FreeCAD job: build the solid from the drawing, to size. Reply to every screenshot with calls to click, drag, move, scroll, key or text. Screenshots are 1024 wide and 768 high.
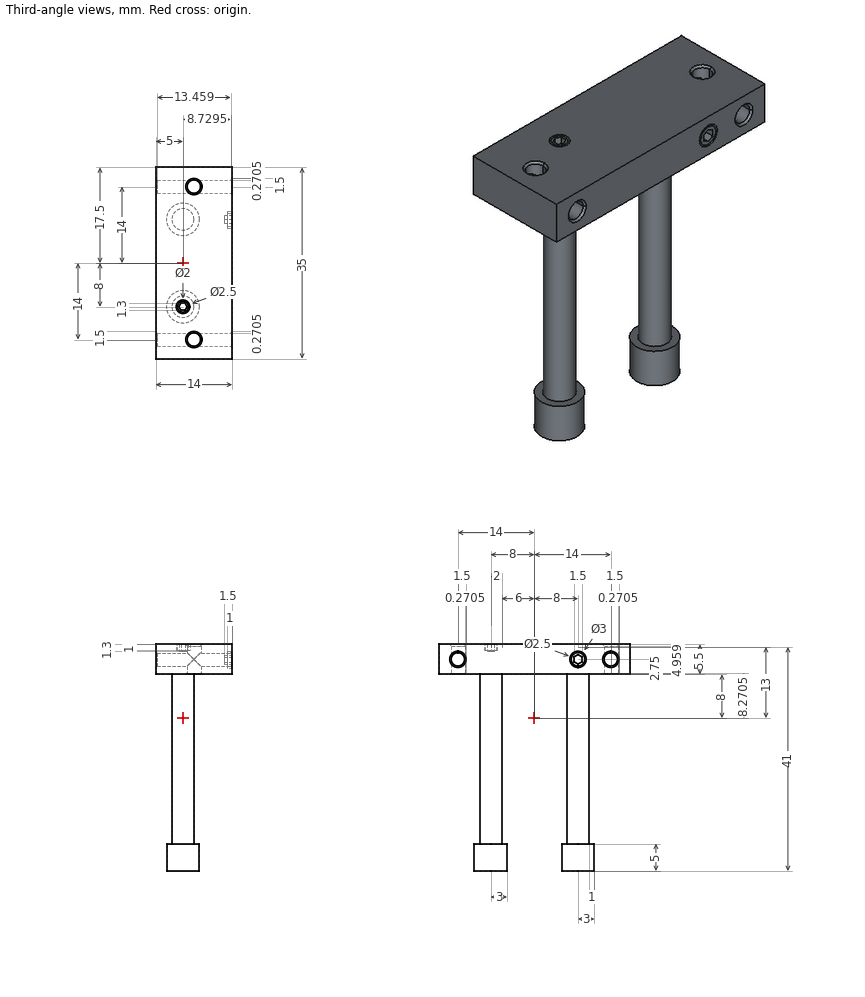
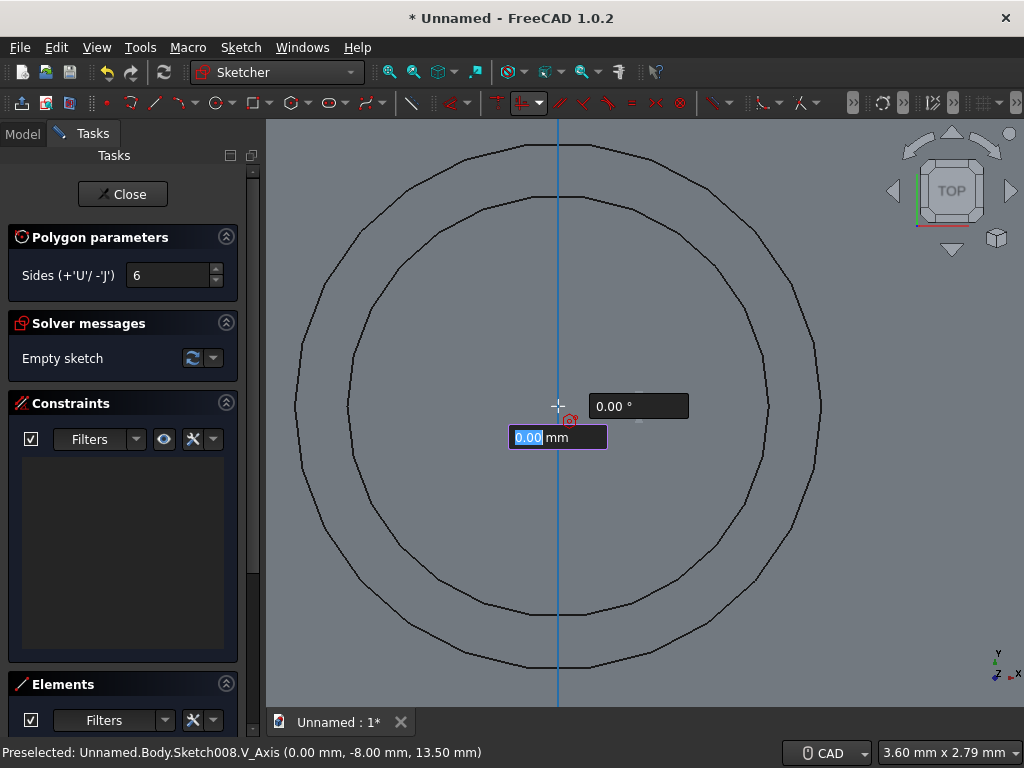
click(400, 406)
right_click(400, 406)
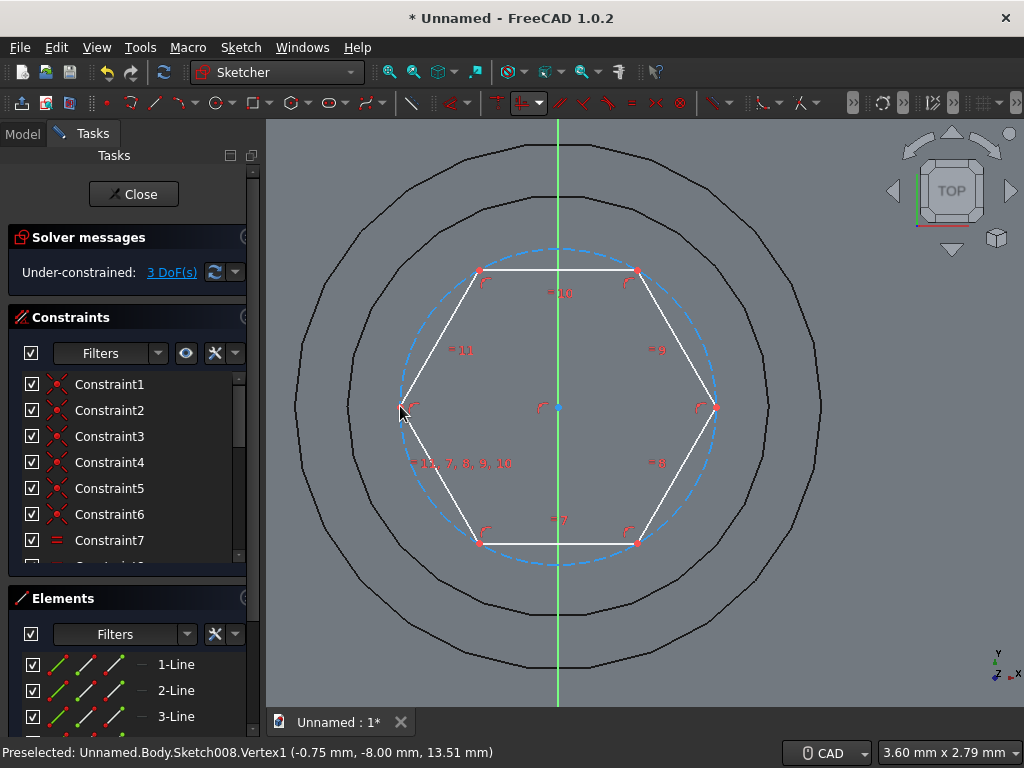
click(527, 544)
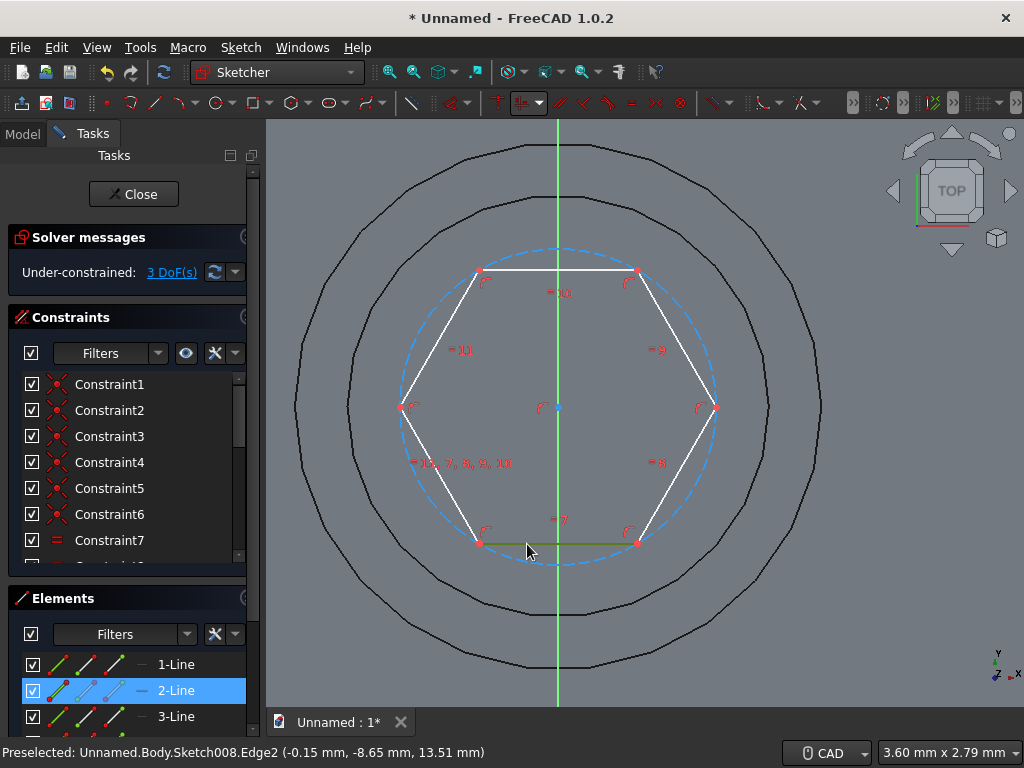
click(542, 104)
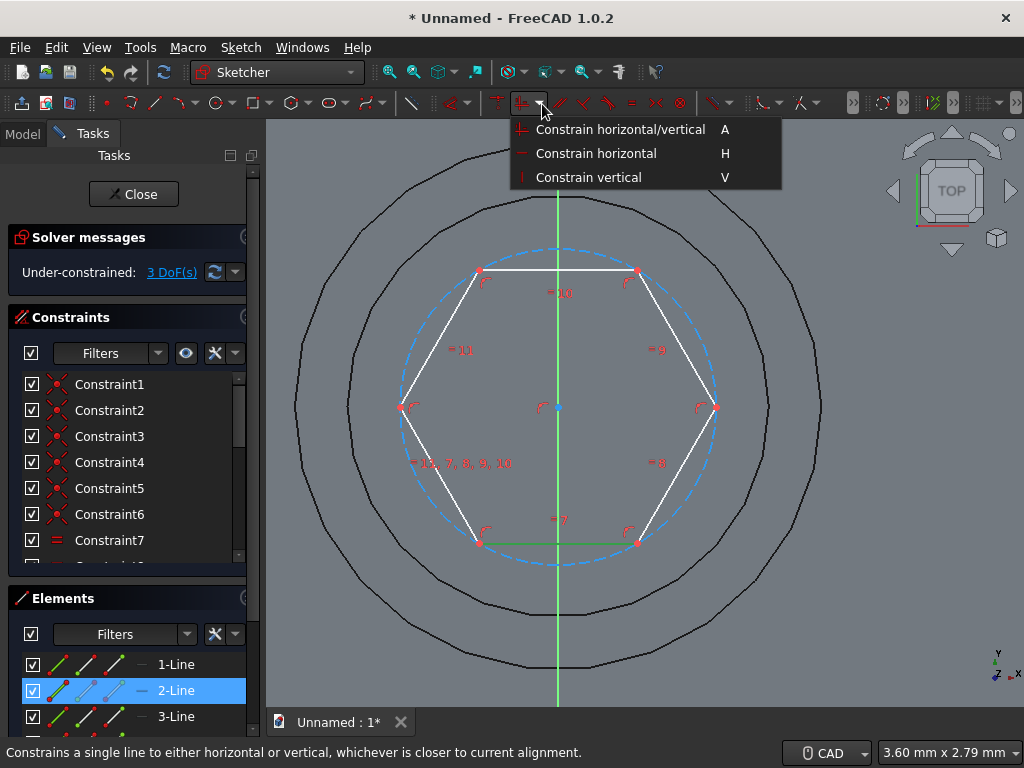
click(646, 153)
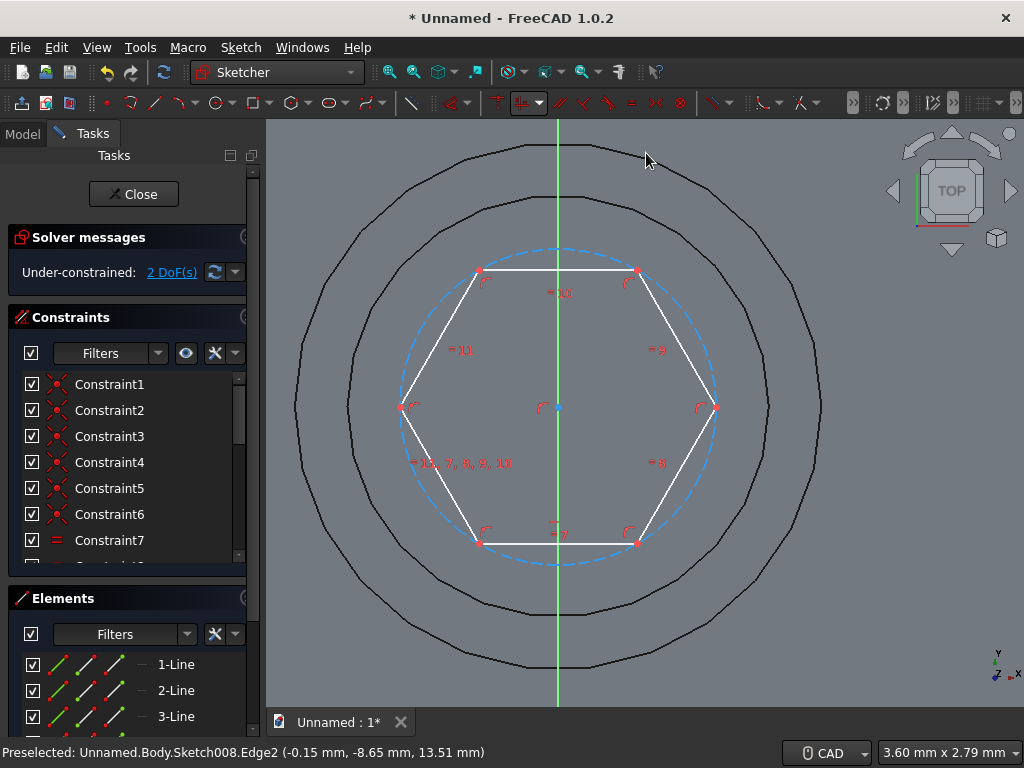
click(450, 104)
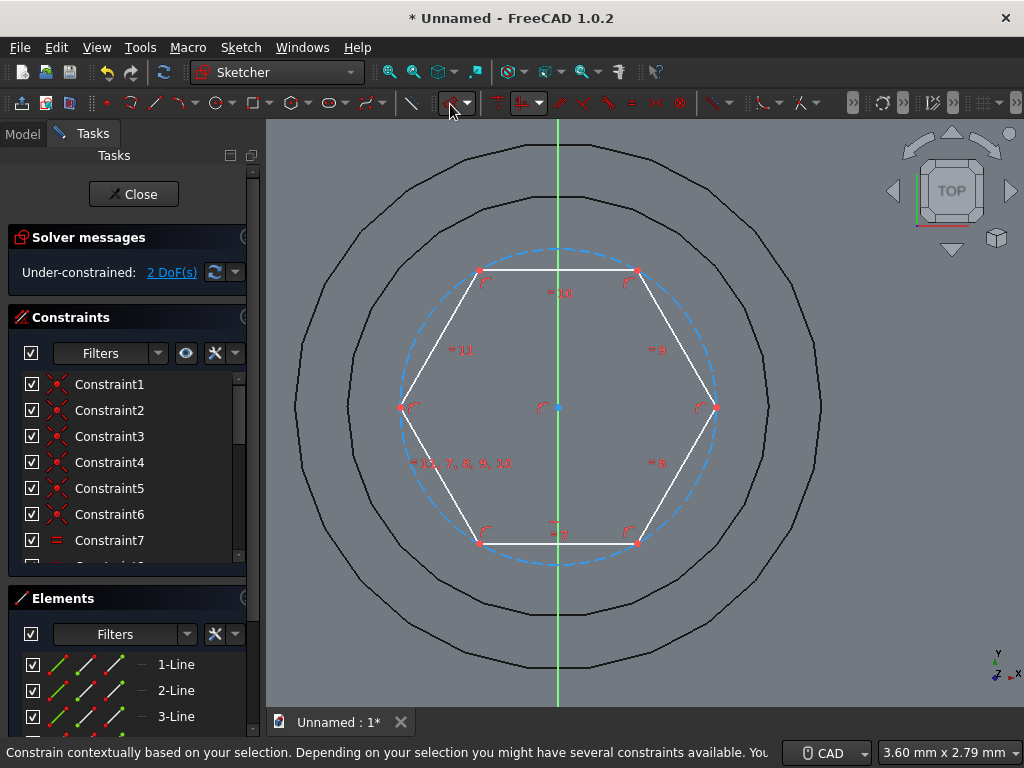
click(558, 407)
click(592, 217)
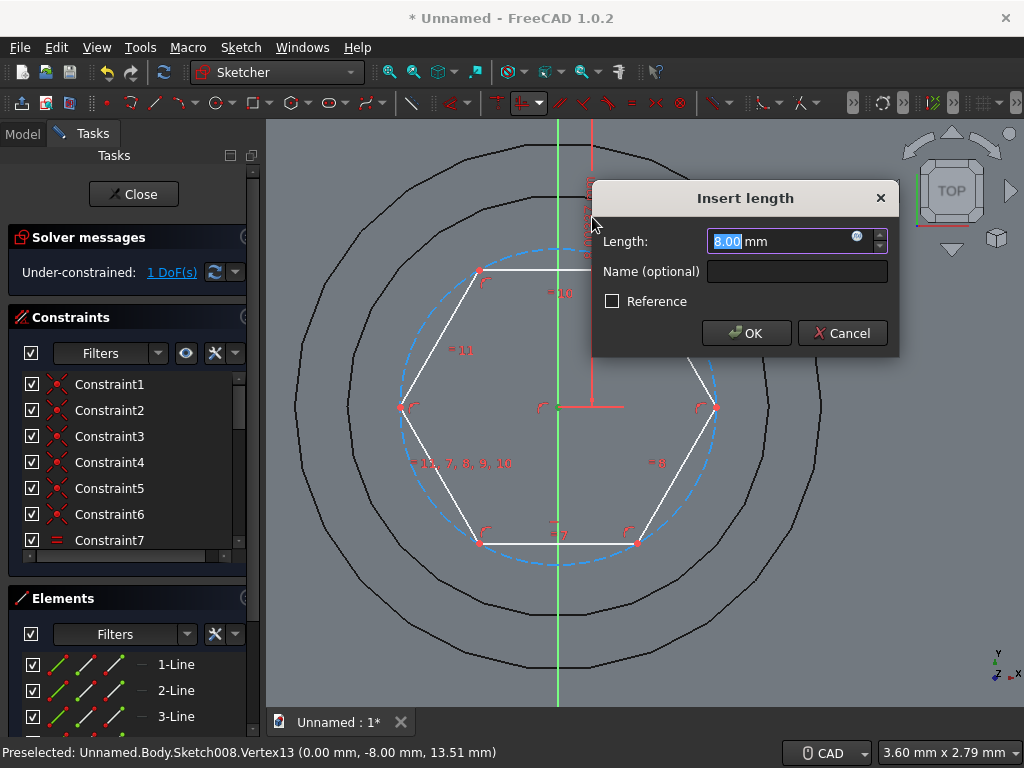
text(8)
key(Return)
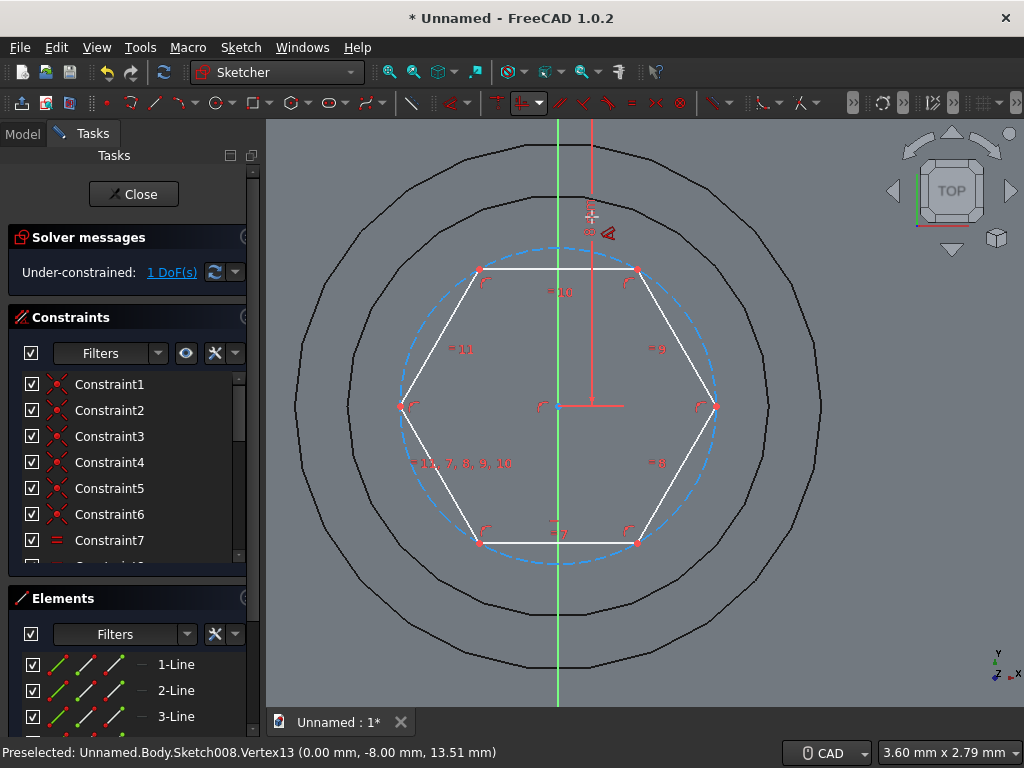
click(479, 543)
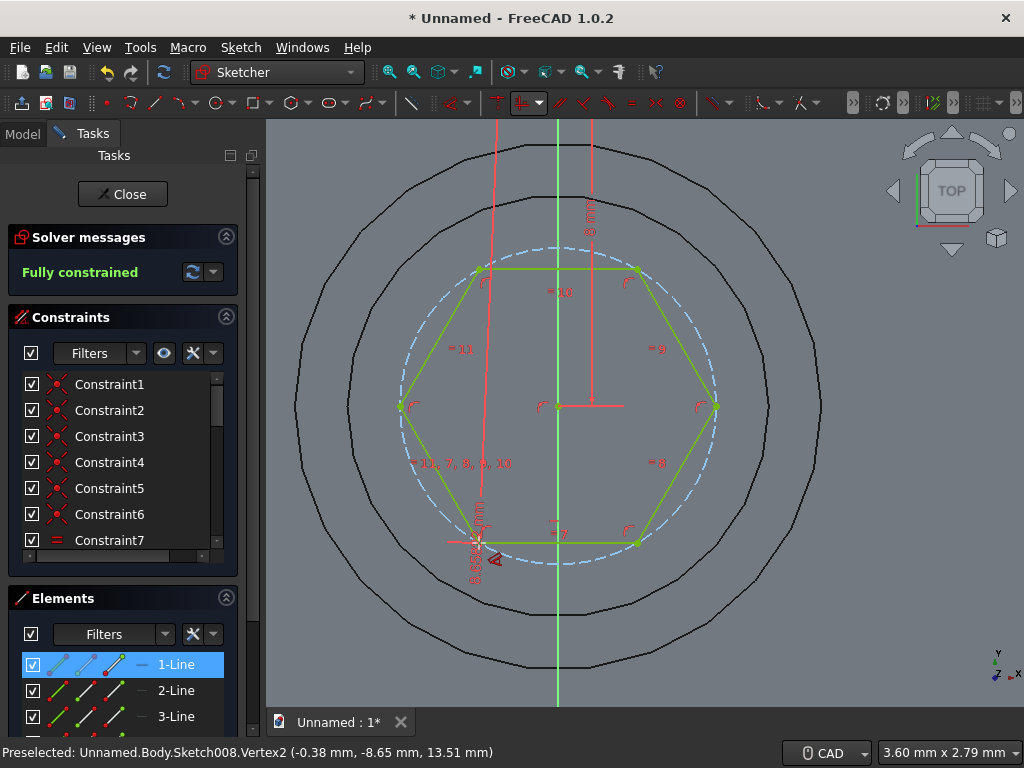
click(637, 269)
click(445, 406)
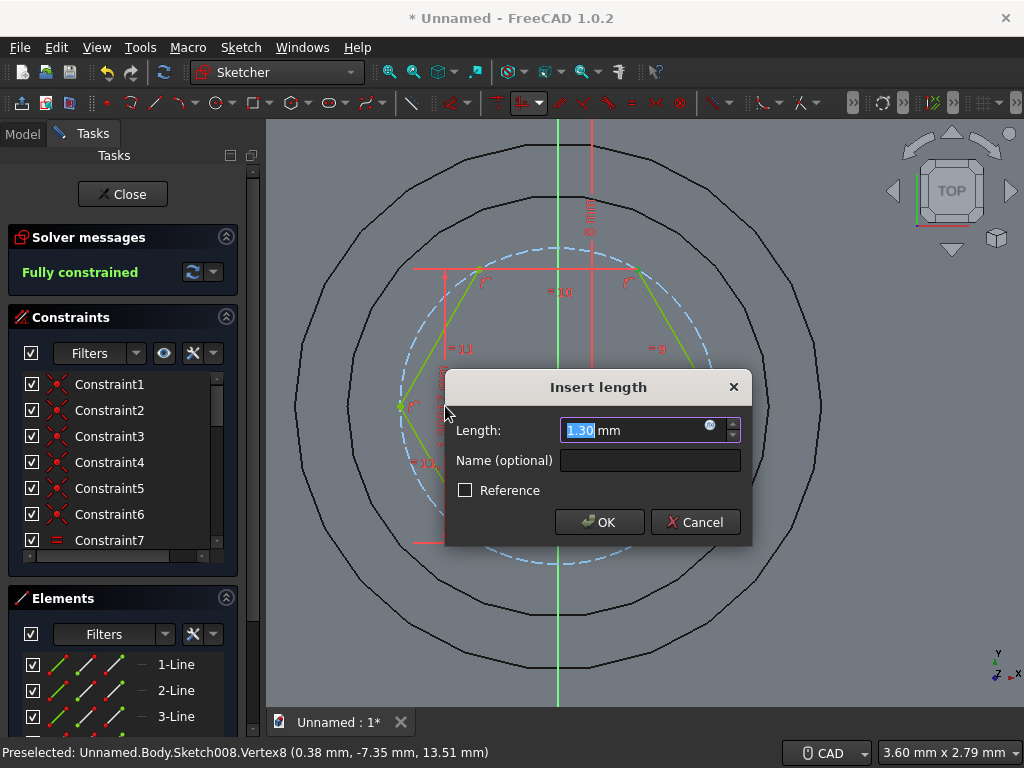
text(1.3)
key(Return)
key(Escape)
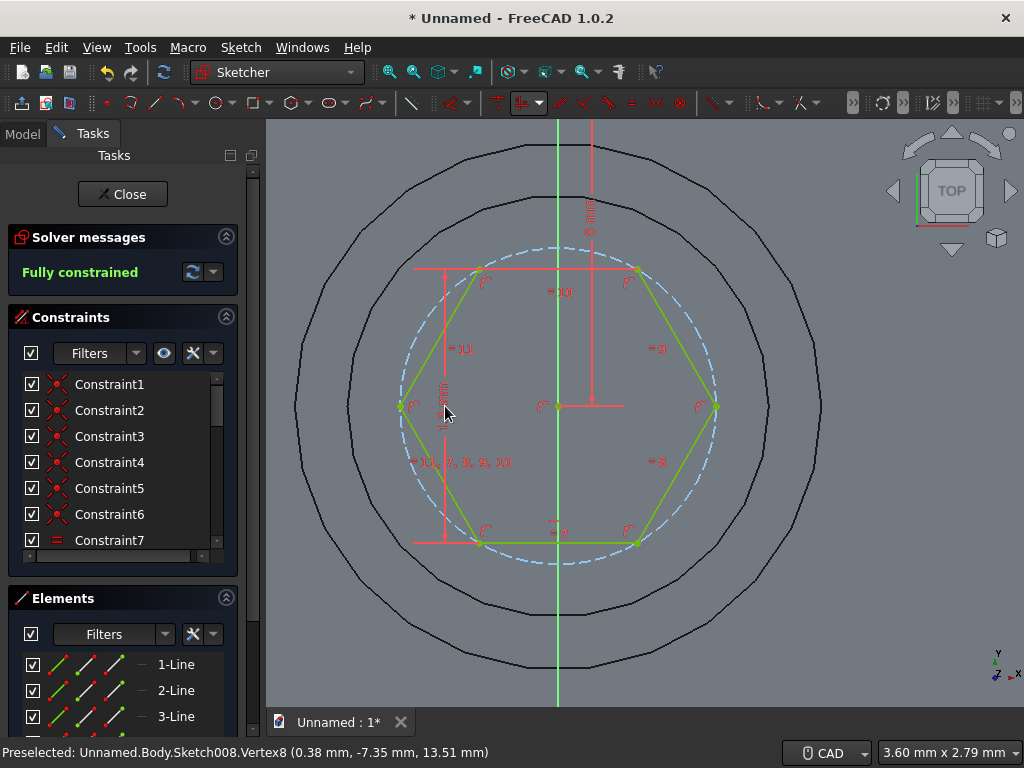
click(123, 194)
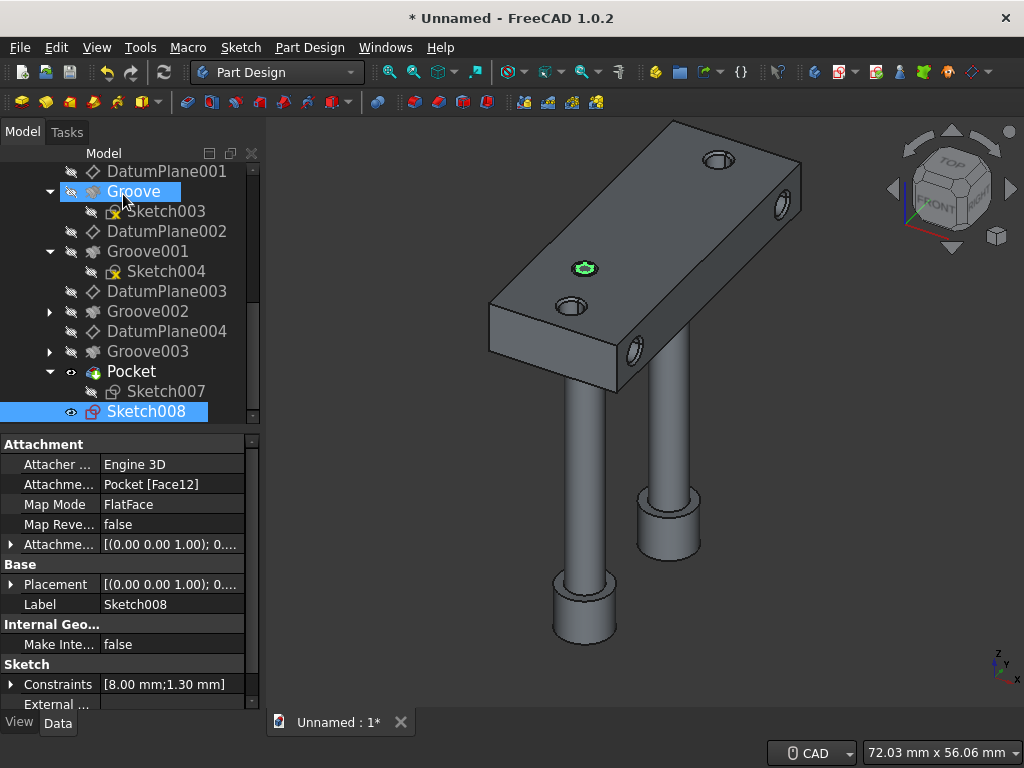
click(188, 102)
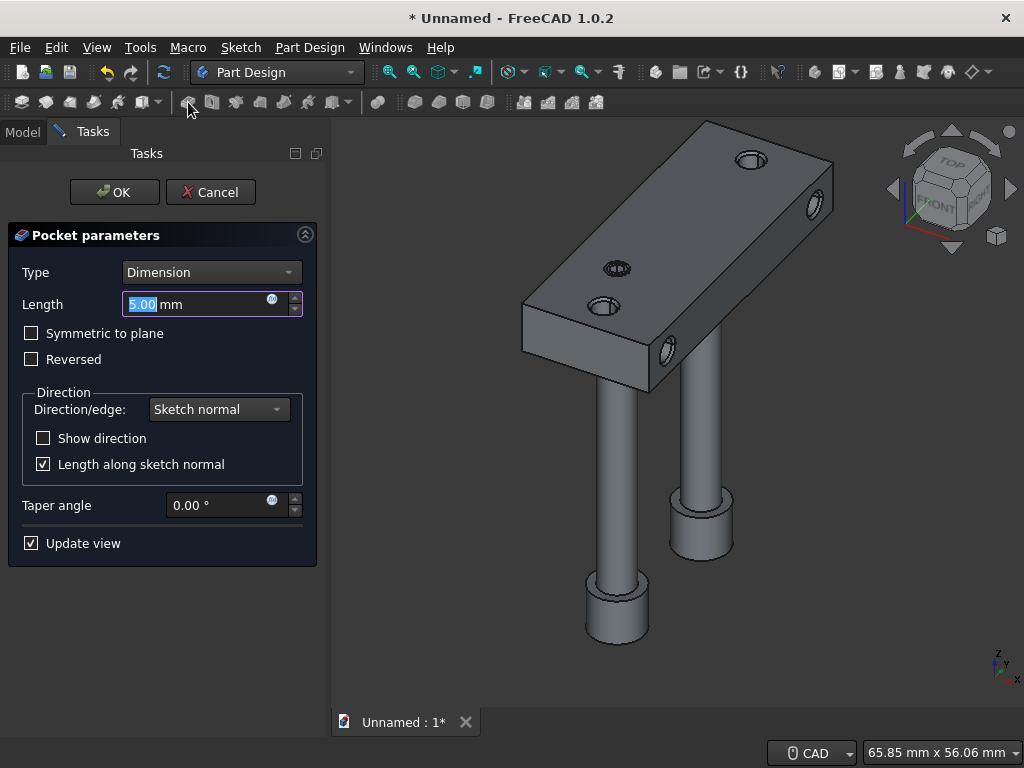
text(1.3)
key(Tab)